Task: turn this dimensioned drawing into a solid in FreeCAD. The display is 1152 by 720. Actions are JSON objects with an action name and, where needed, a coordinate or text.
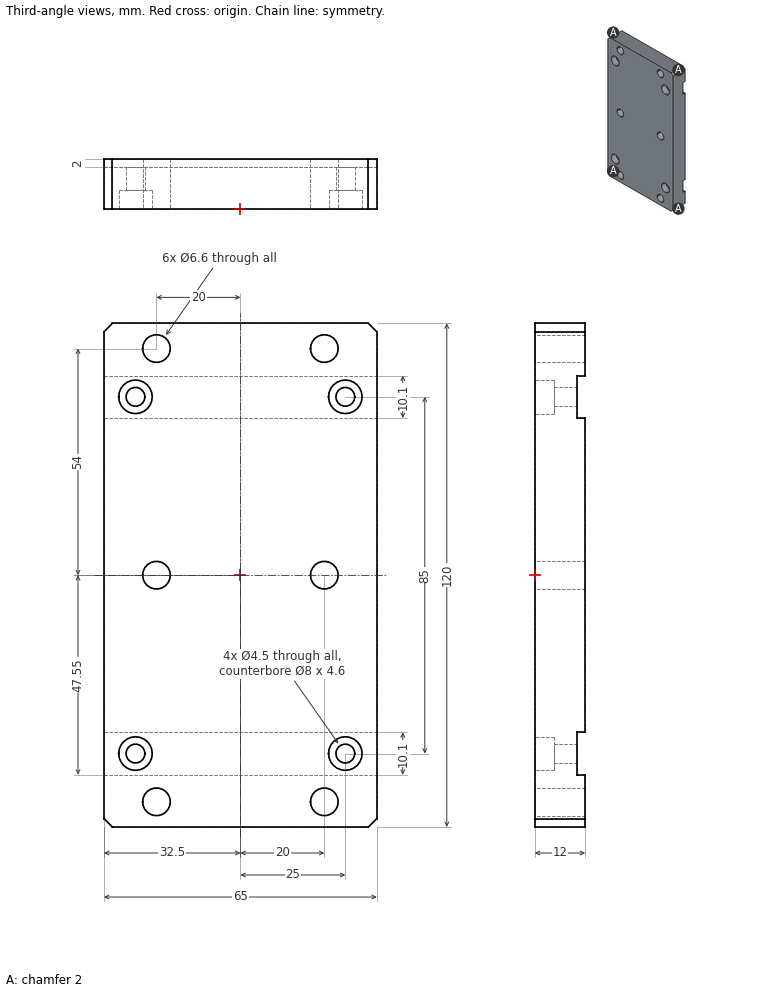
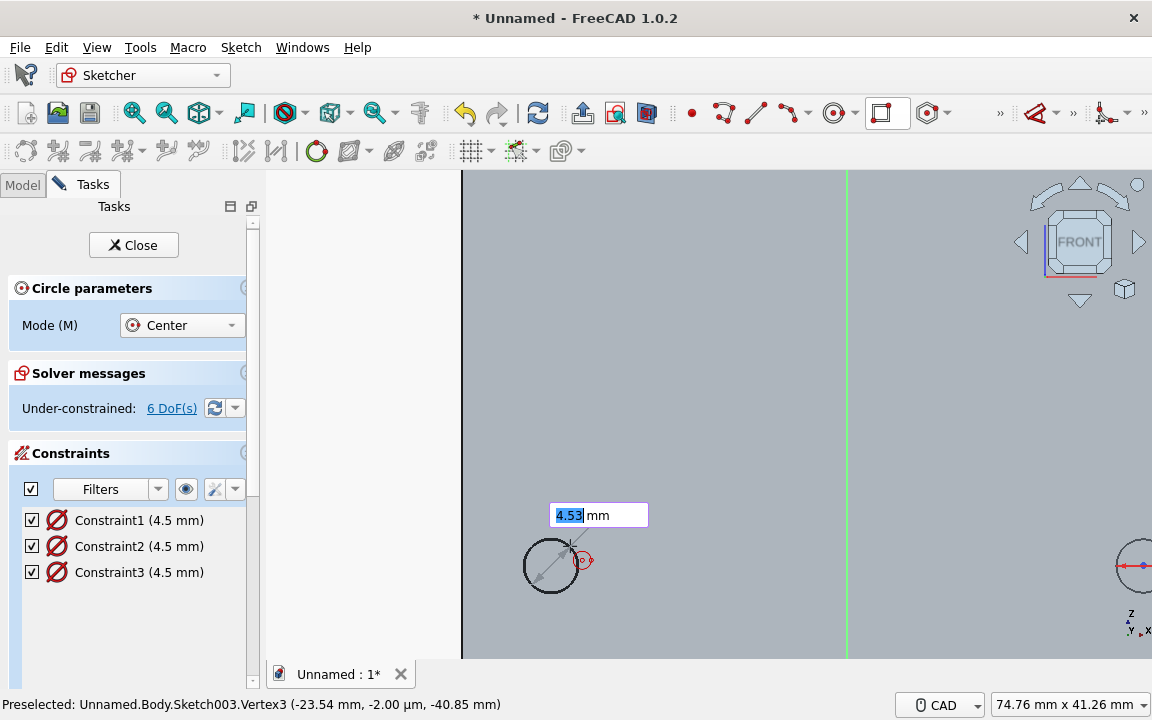
{"action": "type", "text": "4.5"}
{"action": "key", "text": "Return"}
{"action": "key", "text": "Escape"}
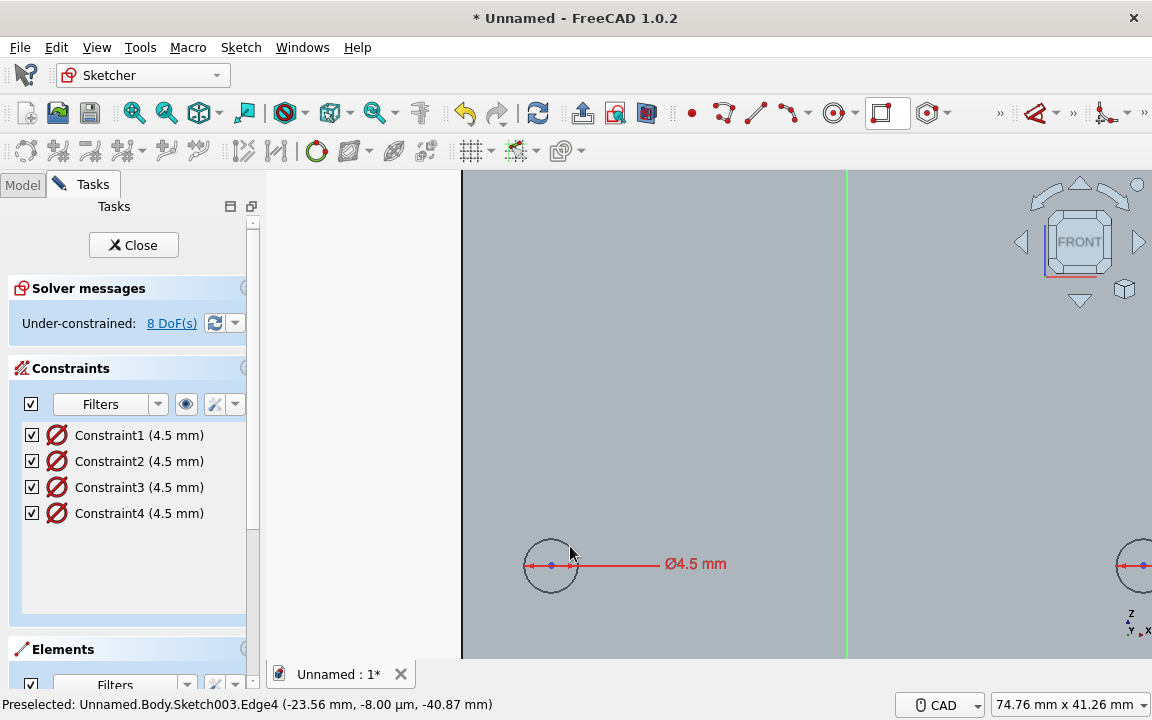
{"action": "scroll", "coordinate": [551, 567], "scroll_direction": "down", "scroll_amount": 6}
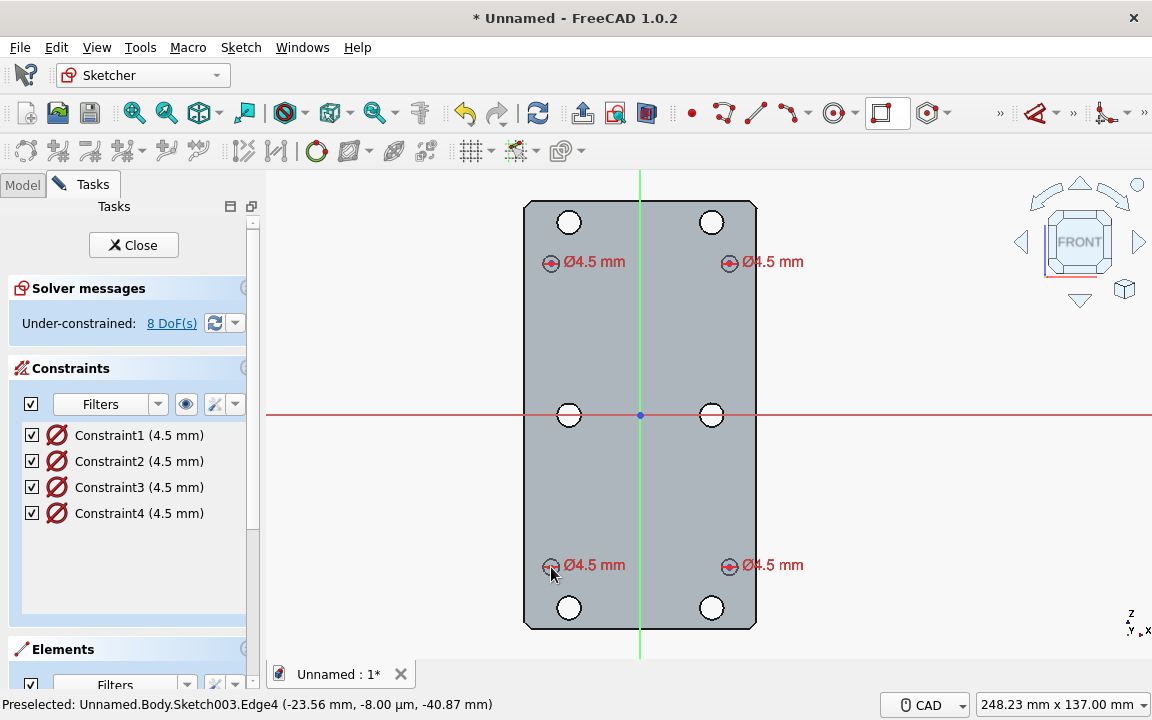
{"action": "left_click", "coordinate": [730, 567]}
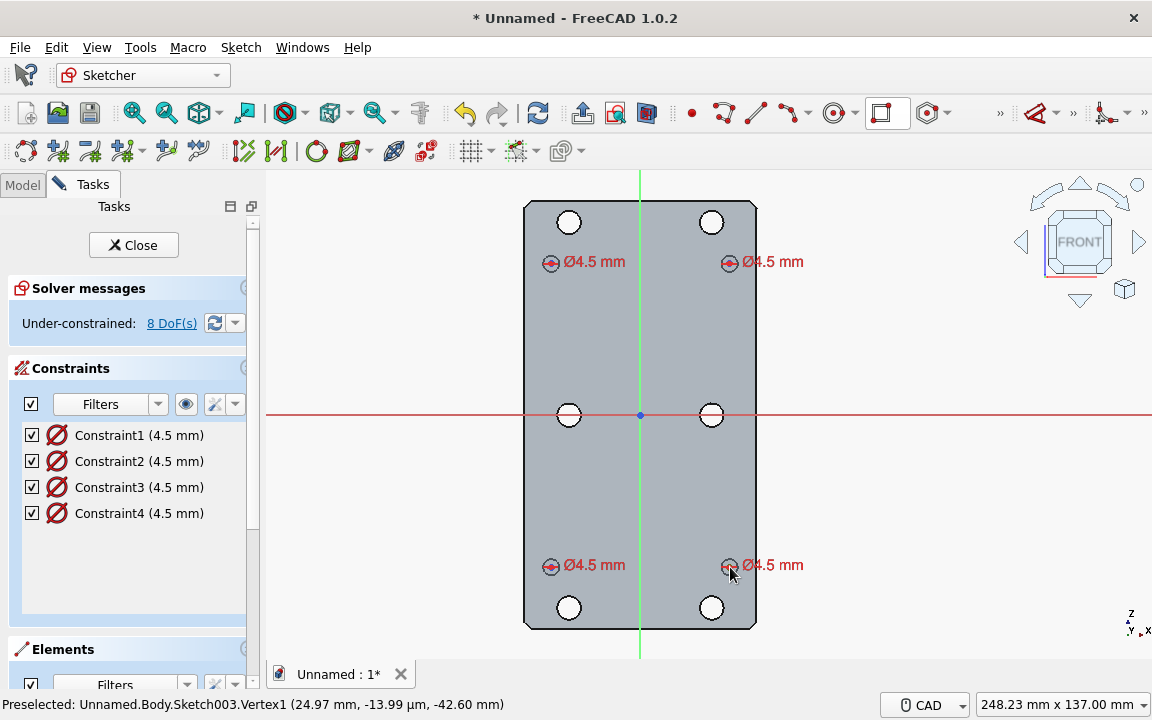
{"action": "left_click", "coordinate": [730, 264]}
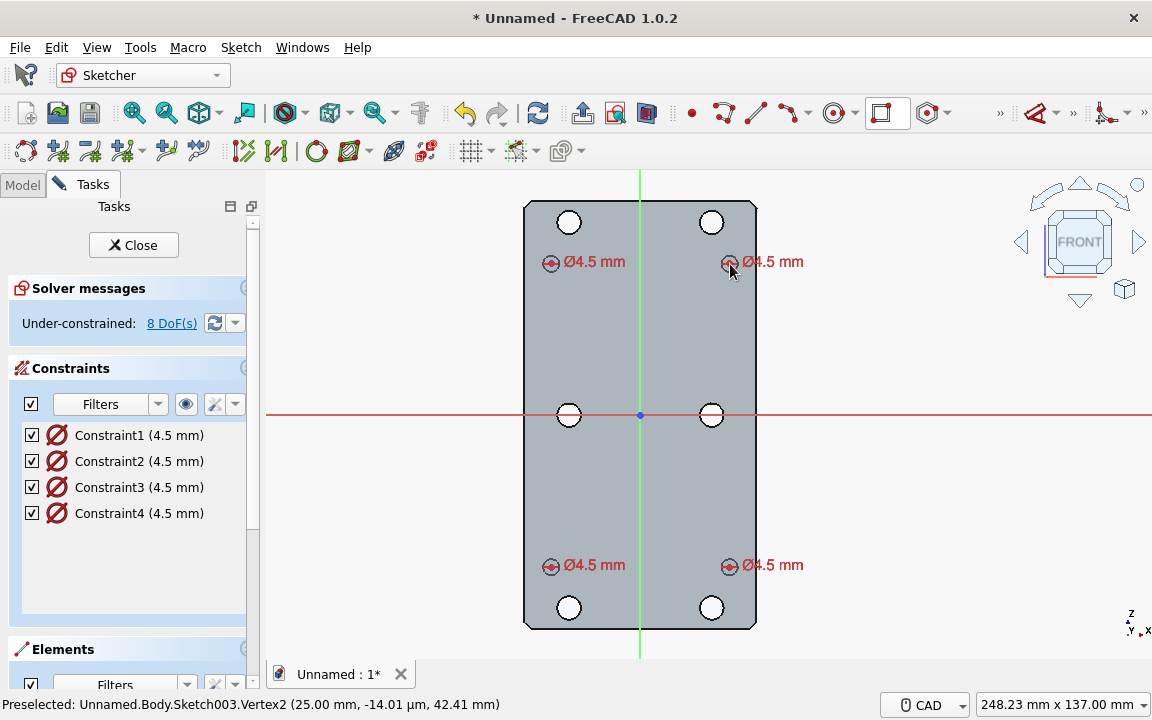
{"action": "left_click", "coordinate": [344, 415]}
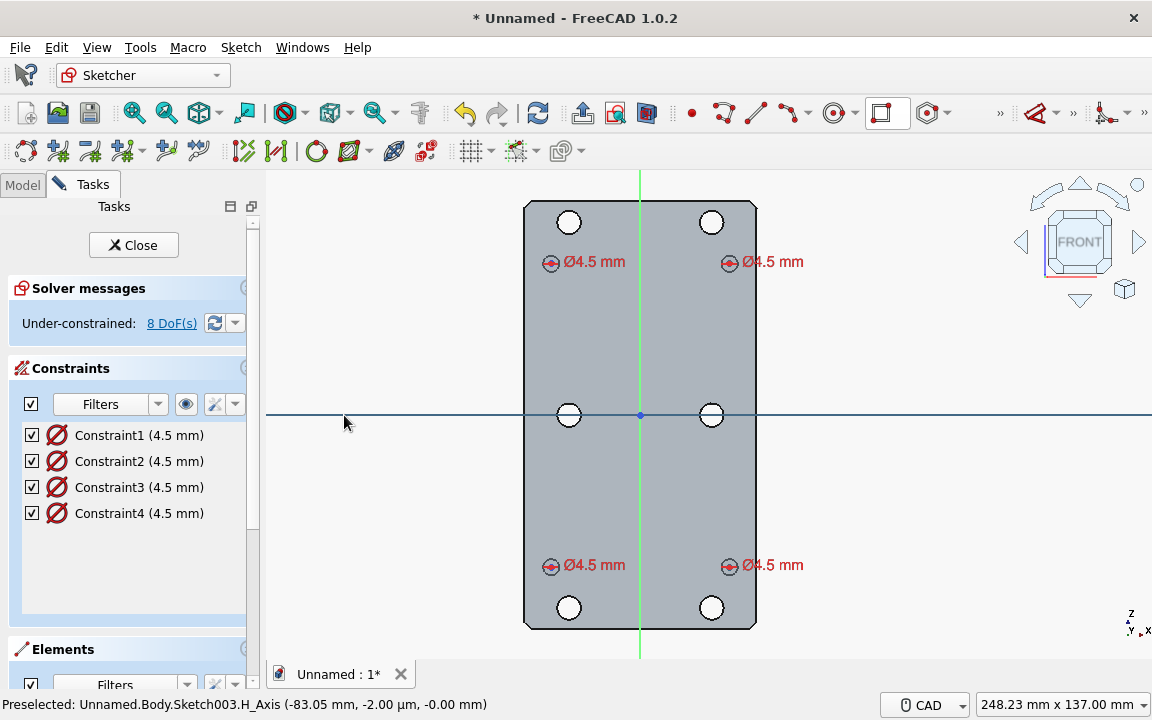
{"action": "key", "text": "s"}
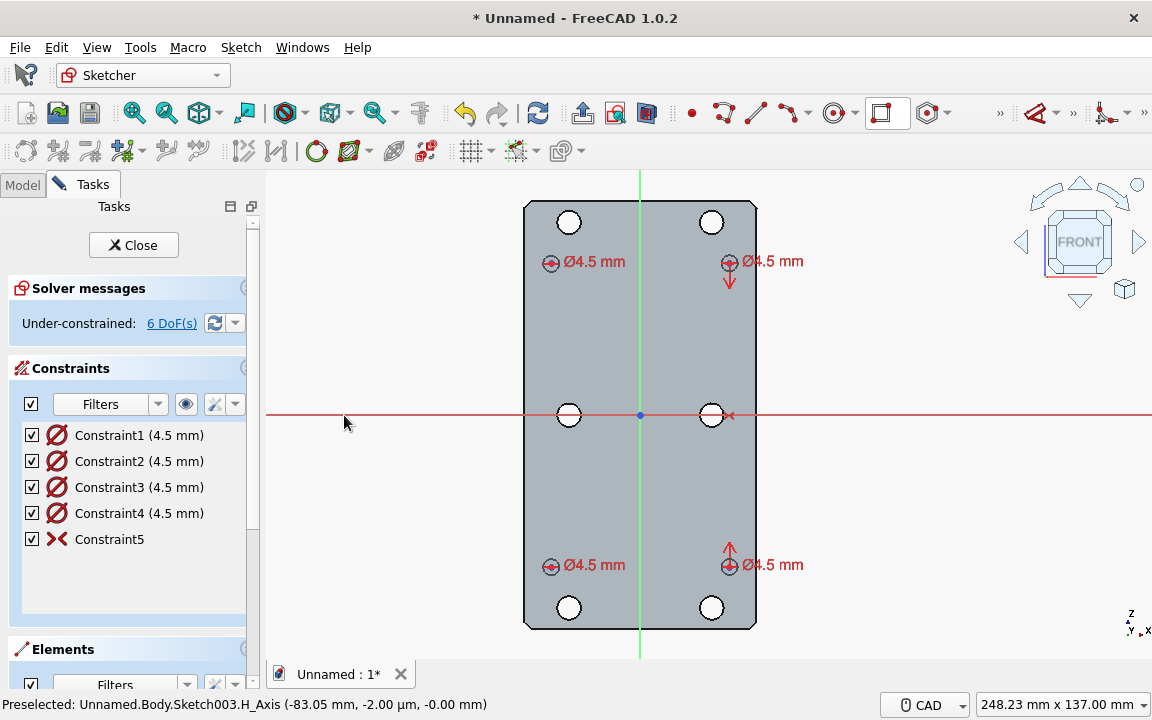
{"action": "left_click", "coordinate": [730, 263]}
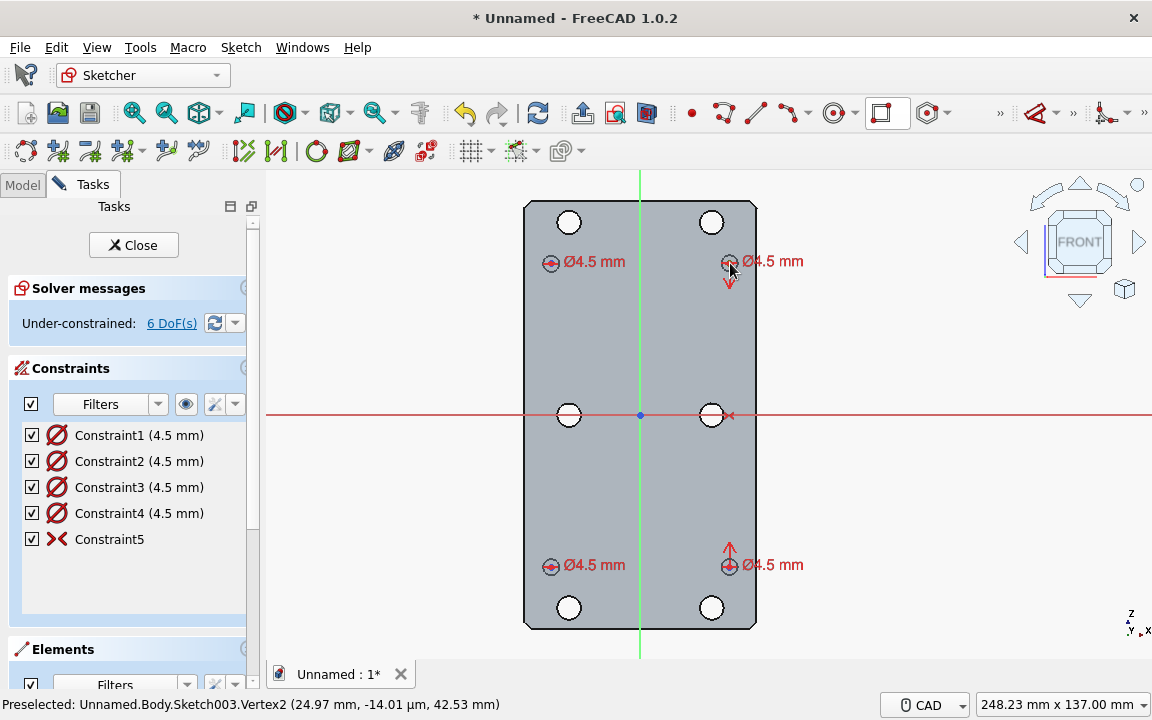
{"action": "left_click", "coordinate": [551, 264]}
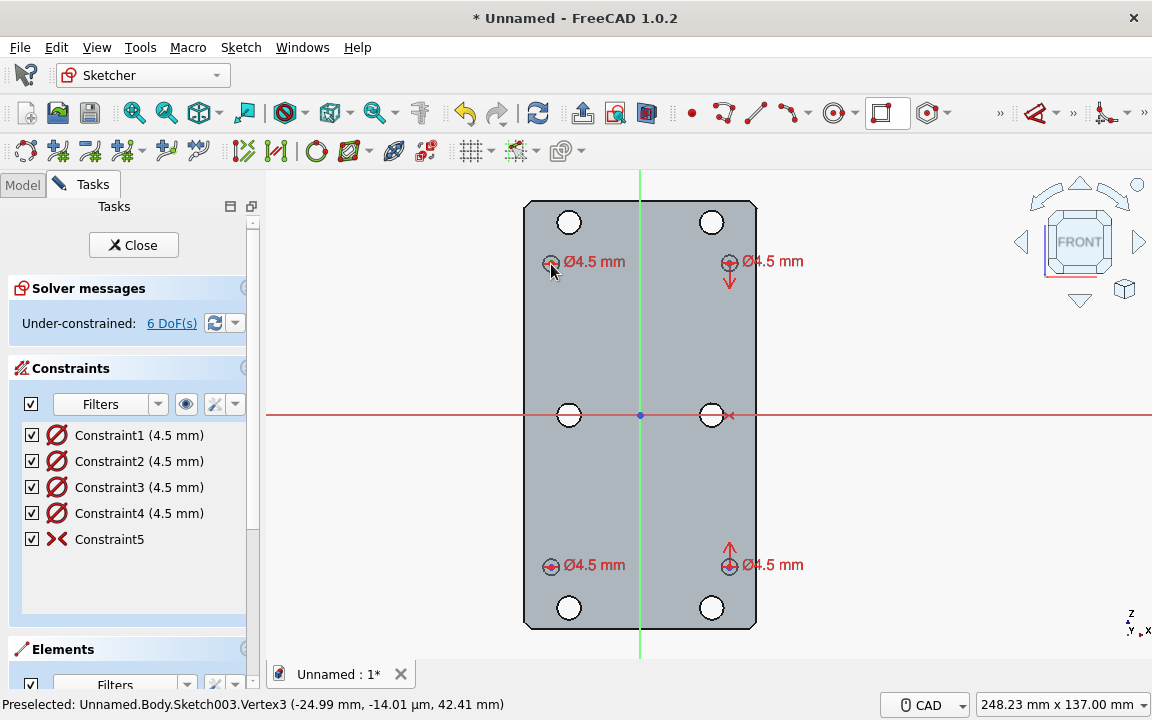
{"action": "left_click", "coordinate": [640, 600]}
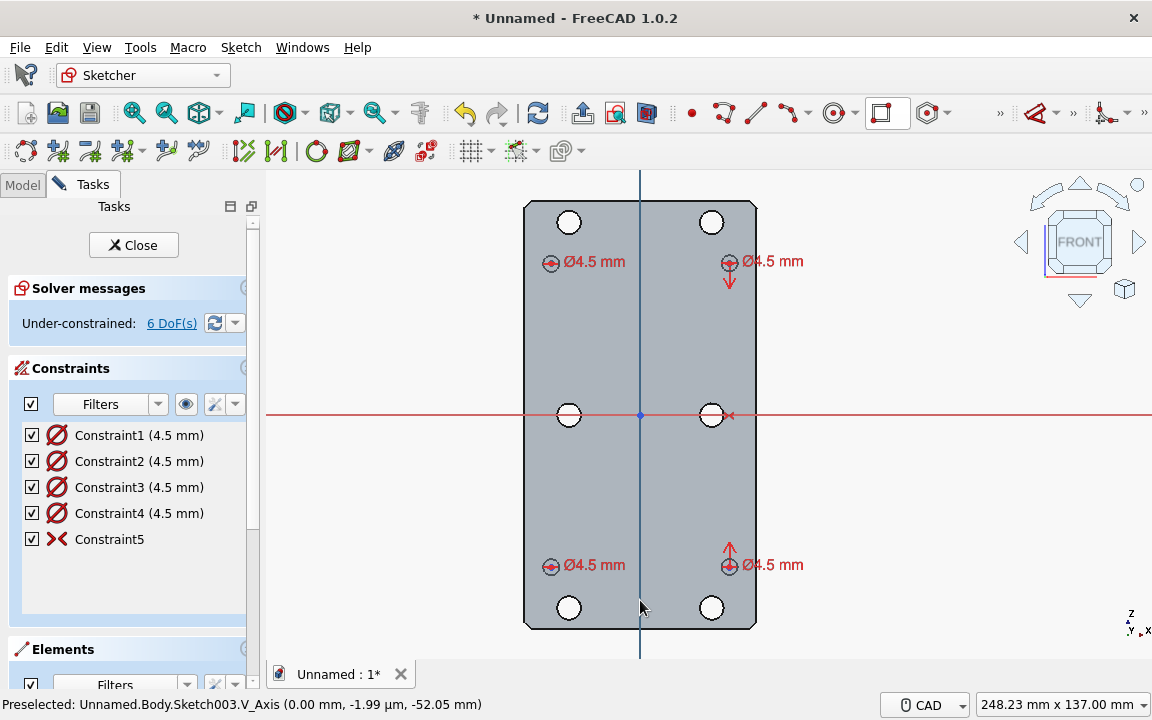
{"action": "key", "text": "s"}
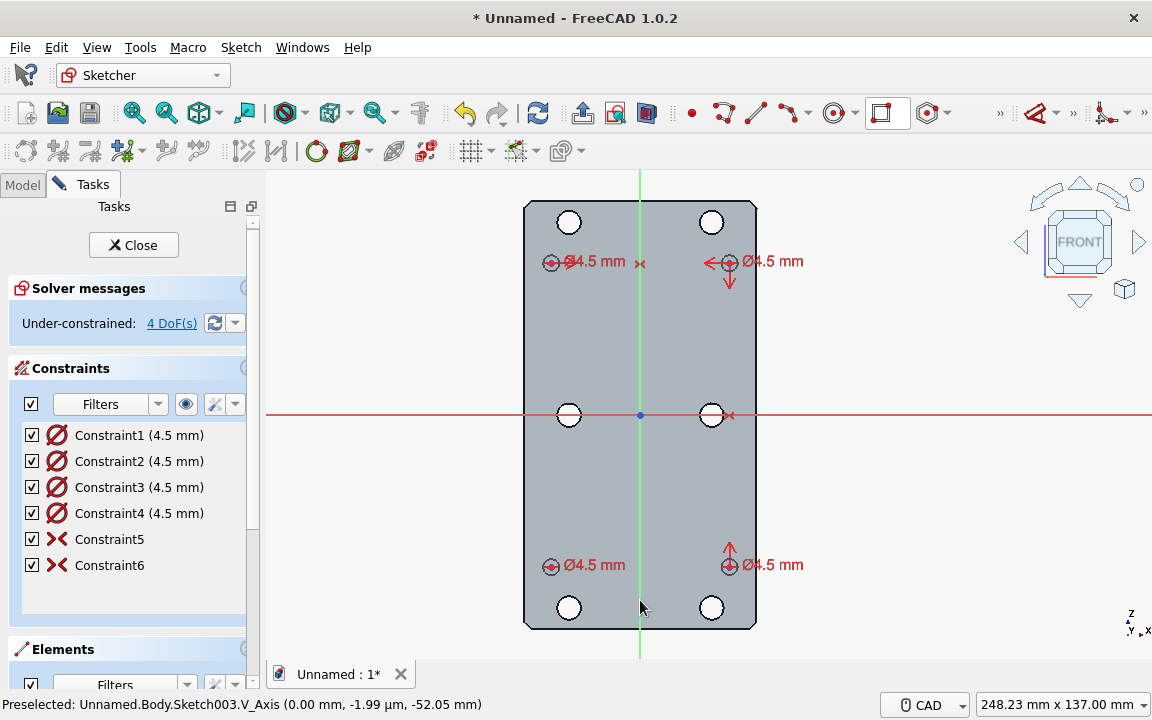
{"action": "left_click", "coordinate": [730, 567]}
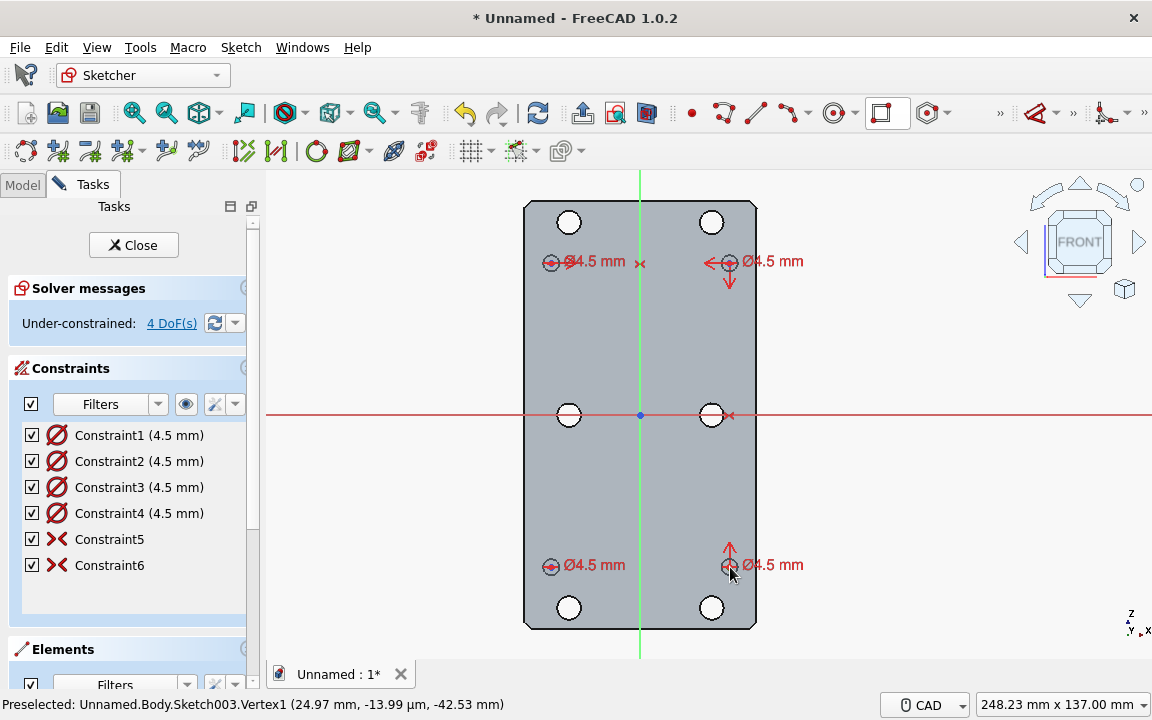
{"action": "left_click", "coordinate": [551, 567]}